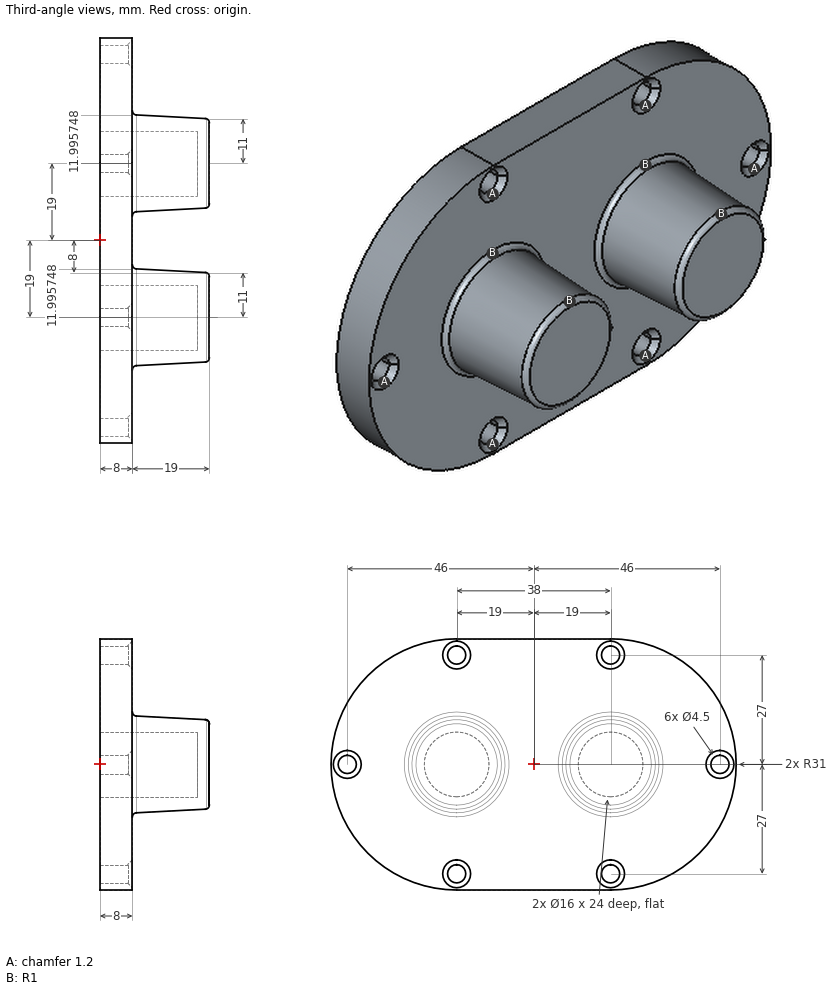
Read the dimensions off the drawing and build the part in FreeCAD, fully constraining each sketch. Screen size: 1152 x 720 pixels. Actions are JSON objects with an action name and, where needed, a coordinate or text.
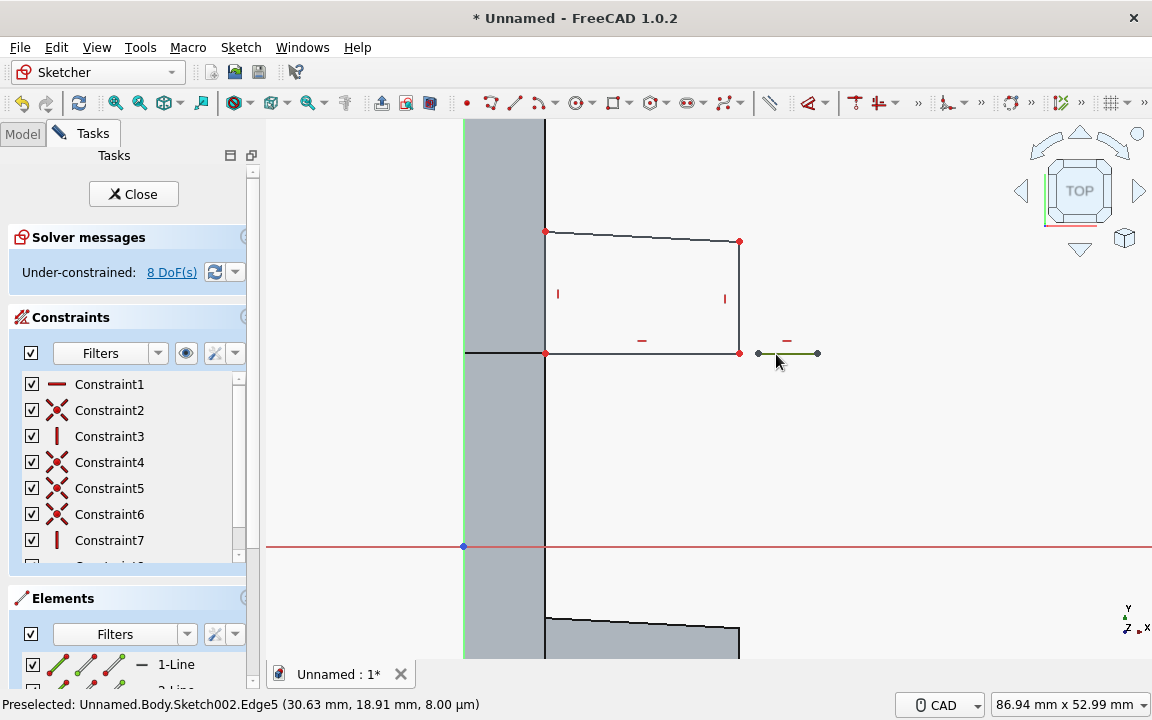
{"action": "left_click", "coordinate": [770, 104]}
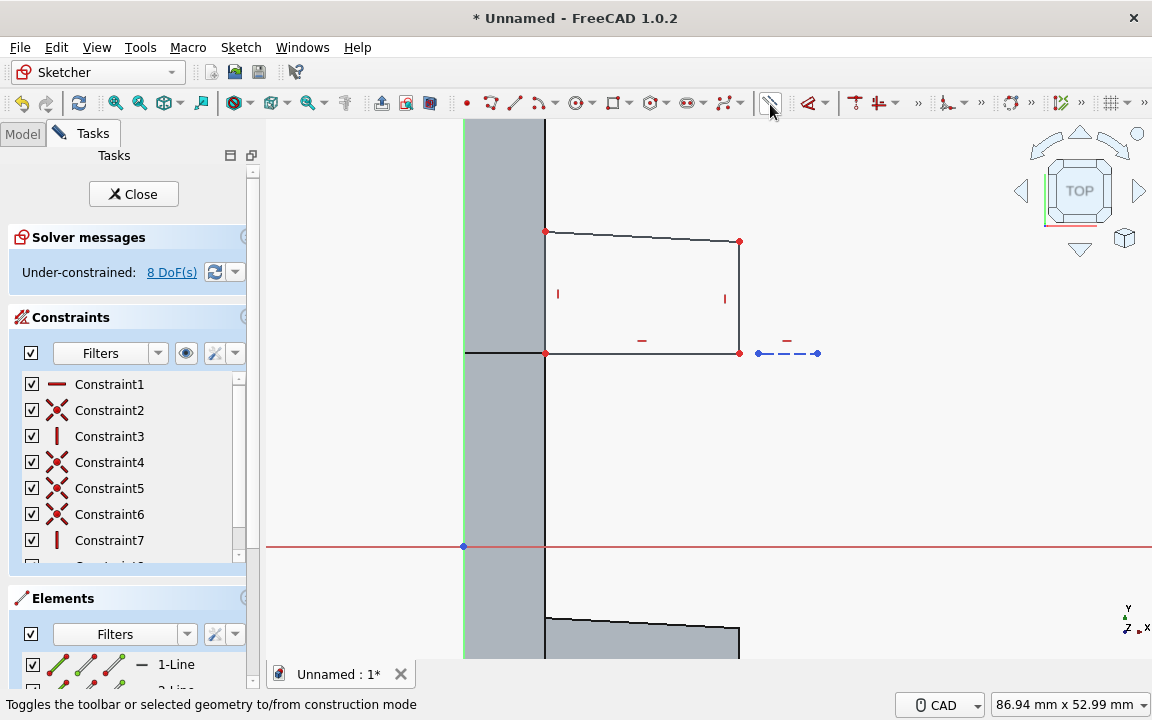
{"action": "left_click", "coordinate": [808, 104]}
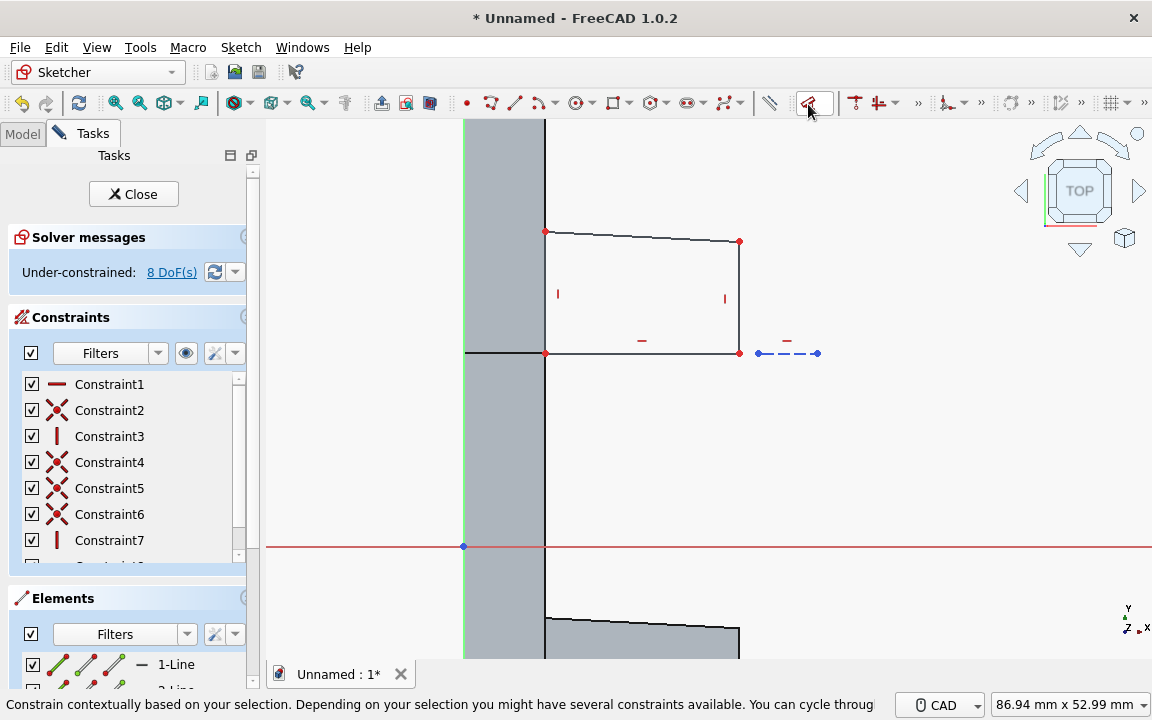
{"action": "left_click", "coordinate": [603, 354]}
{"action": "left_click", "coordinate": [642, 320]}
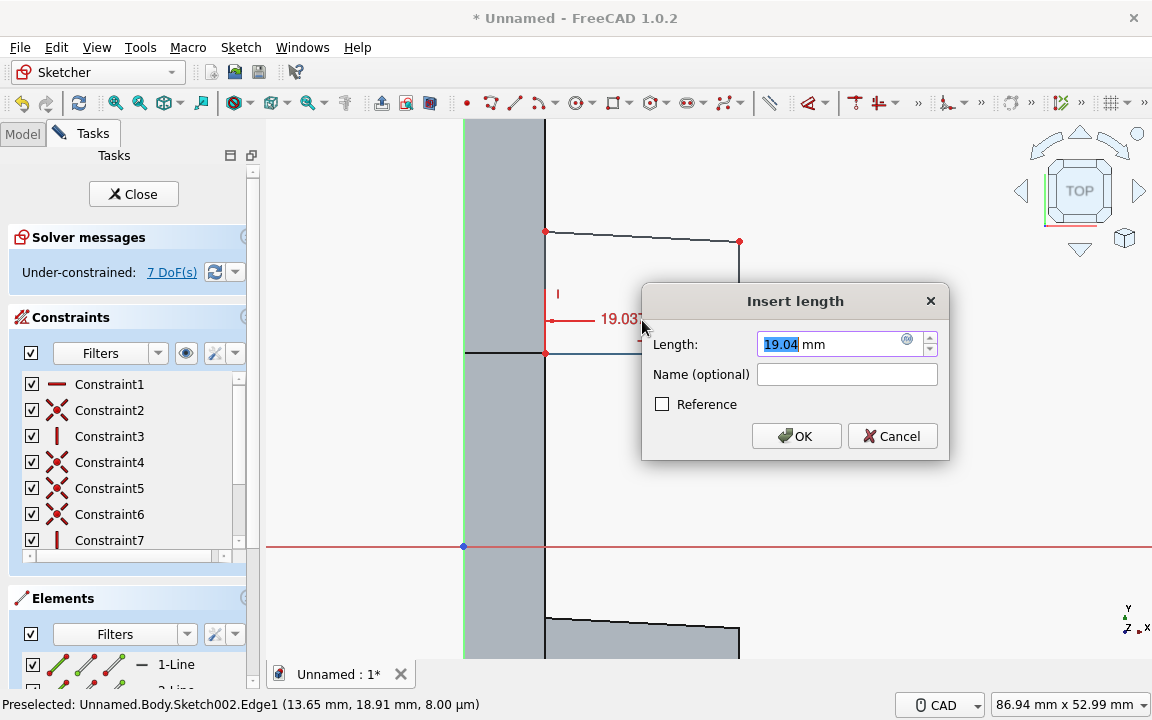
{"action": "type", "text": "19"}
{"action": "key", "text": "Return"}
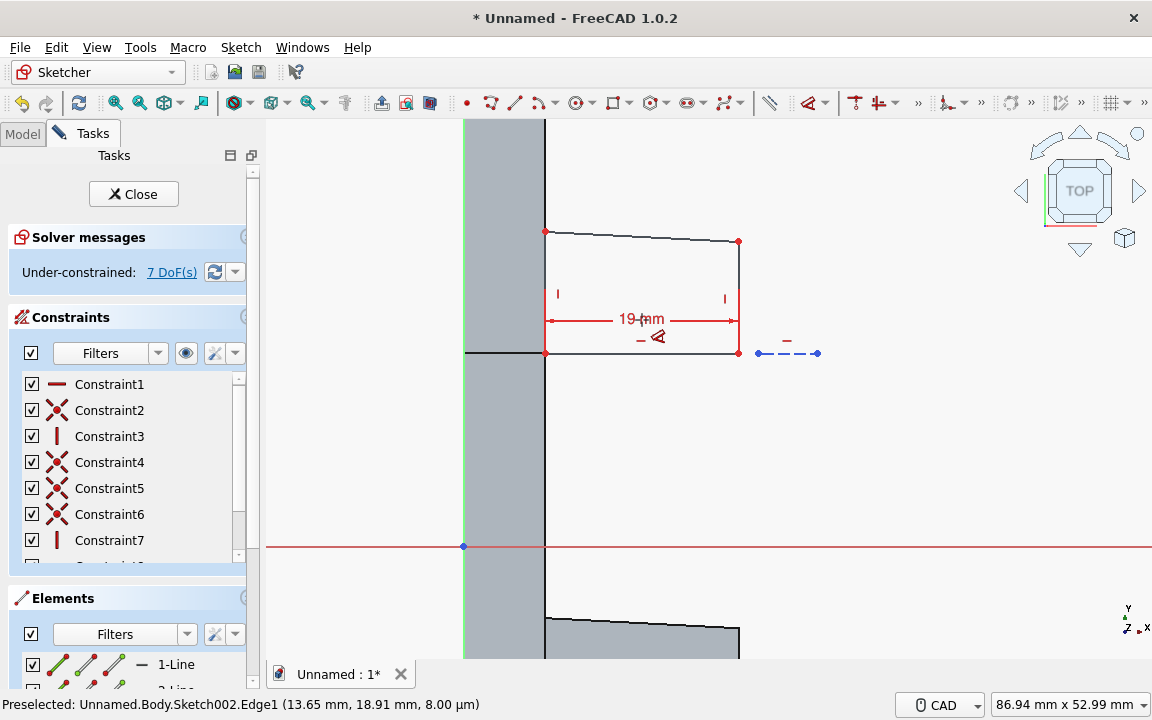
{"action": "left_click", "coordinate": [739, 320]}
{"action": "left_click", "coordinate": [773, 298]}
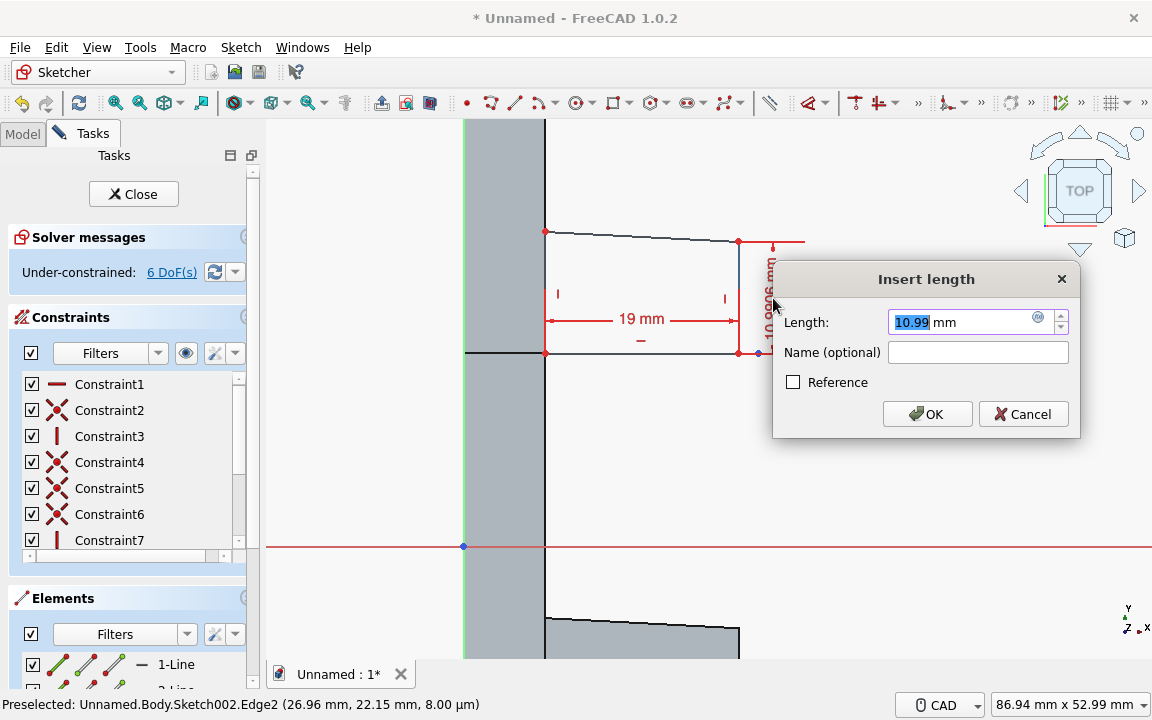
{"action": "type", "text": "11"}
{"action": "key", "text": "Return"}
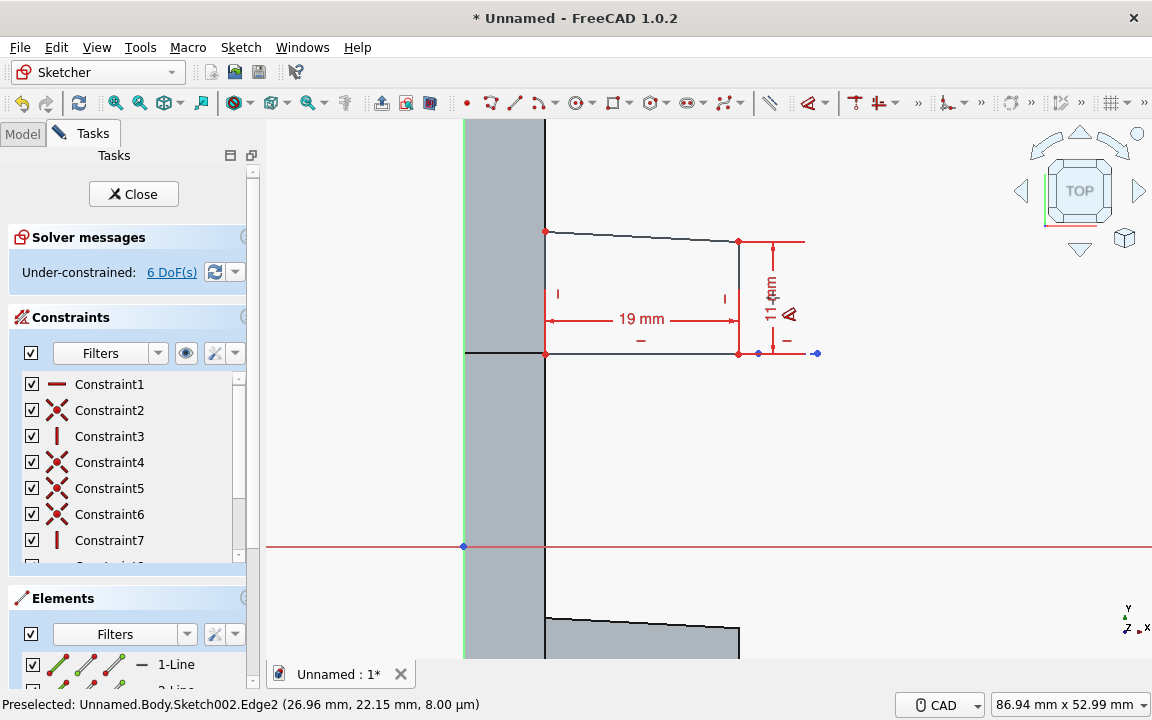
{"action": "left_click", "coordinate": [545, 354]}
{"action": "left_click", "coordinate": [504, 581]}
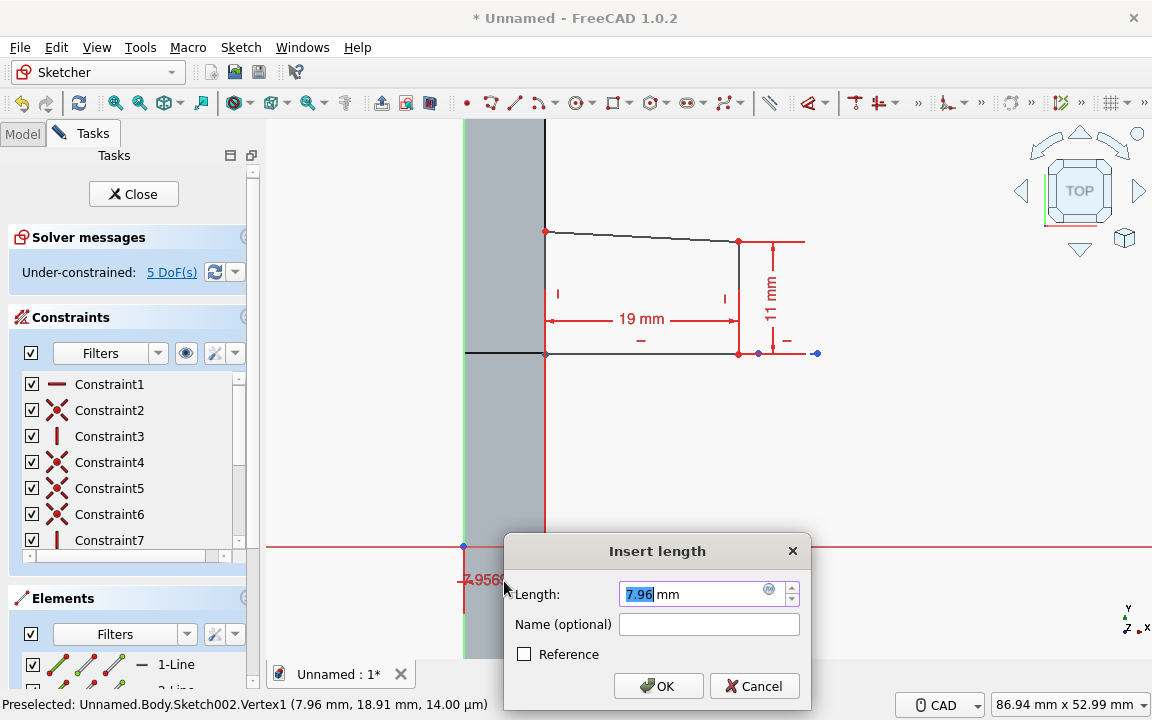
{"action": "type", "text": "8"}
{"action": "key", "text": "Return"}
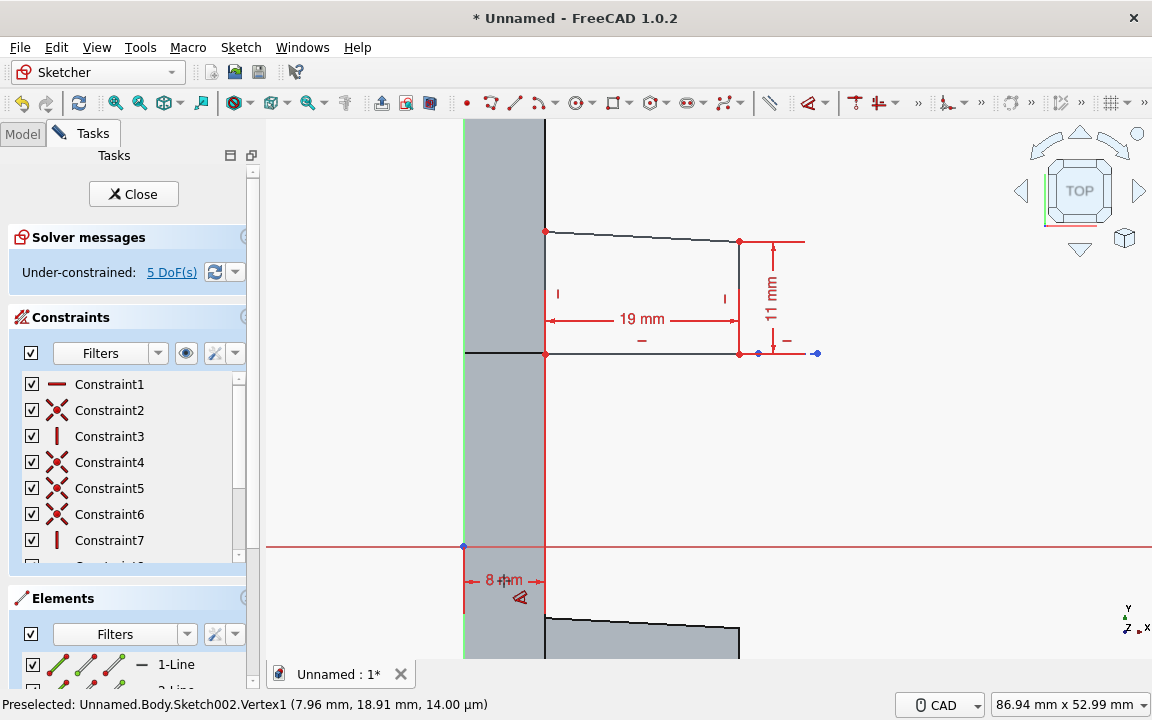
{"action": "left_click", "coordinate": [545, 354]}
{"action": "left_click", "coordinate": [430, 450]}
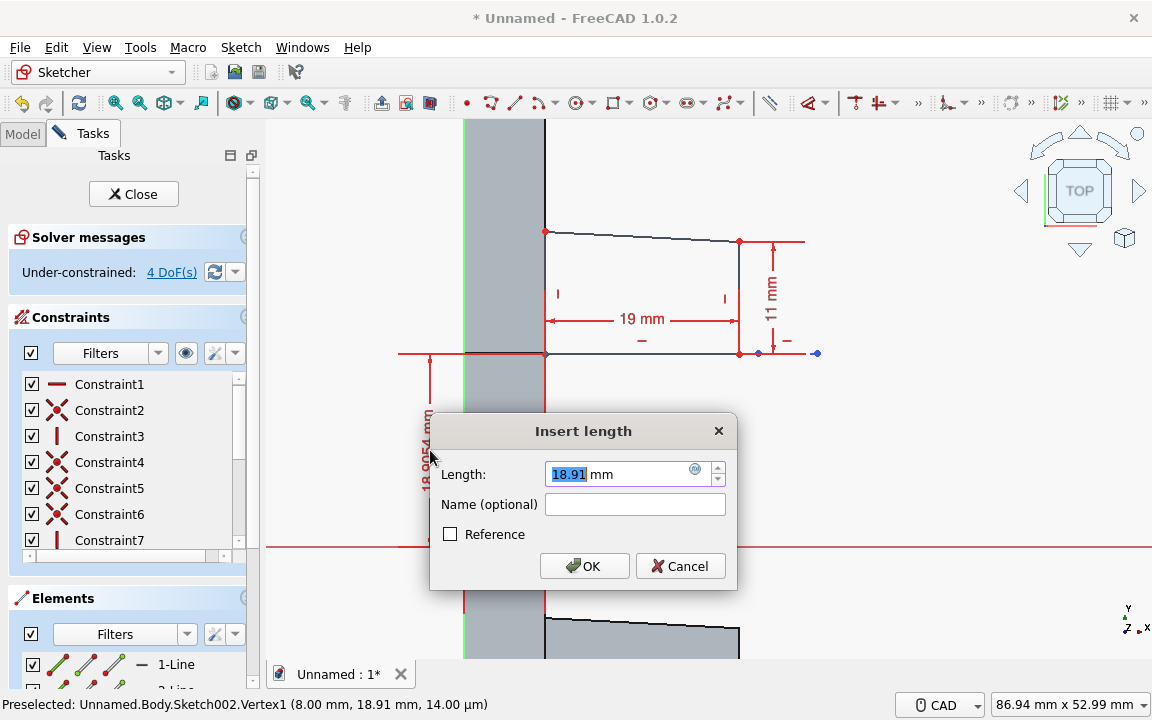
{"action": "type", "text": "19"}
{"action": "key", "text": "Return"}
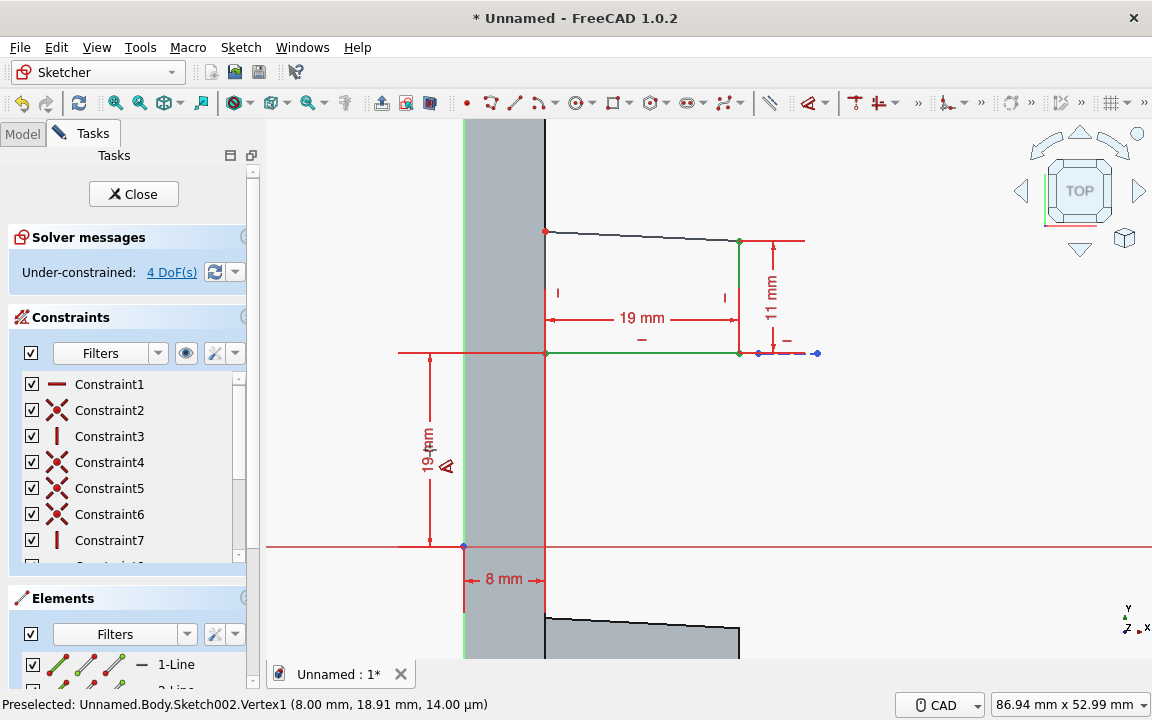
{"action": "left_click", "coordinate": [758, 354]}
{"action": "left_click", "coordinate": [430, 406]}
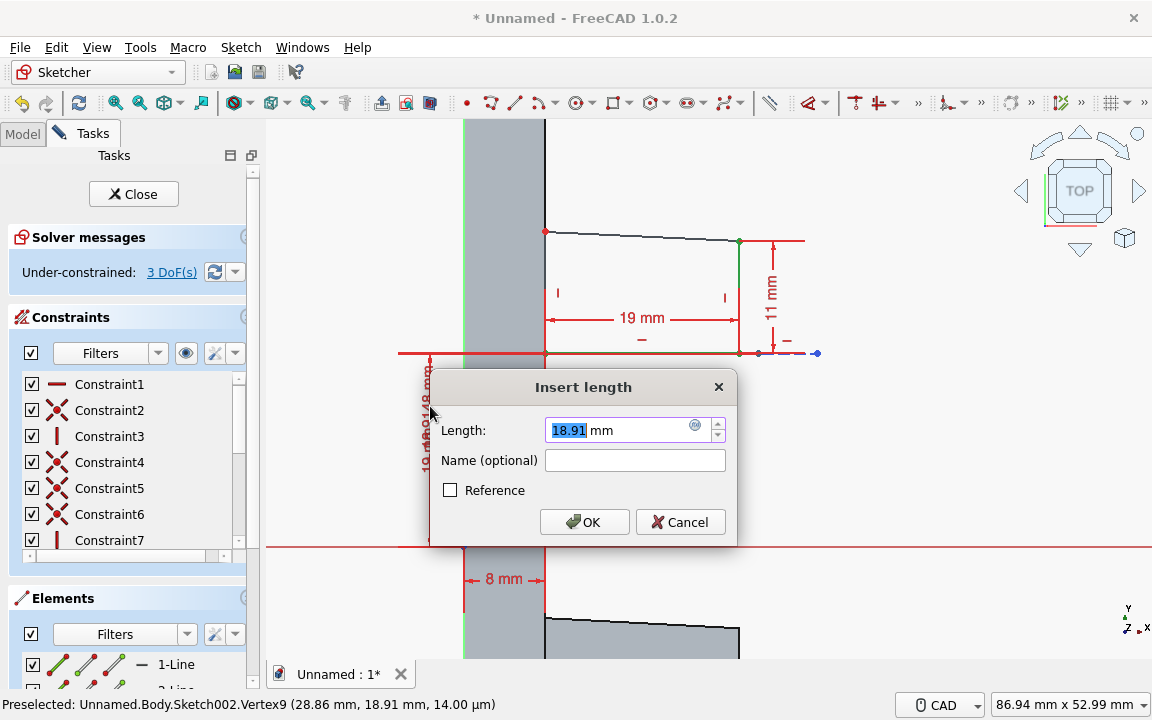
{"action": "type", "text": "19"}
{"action": "key", "text": "Return"}